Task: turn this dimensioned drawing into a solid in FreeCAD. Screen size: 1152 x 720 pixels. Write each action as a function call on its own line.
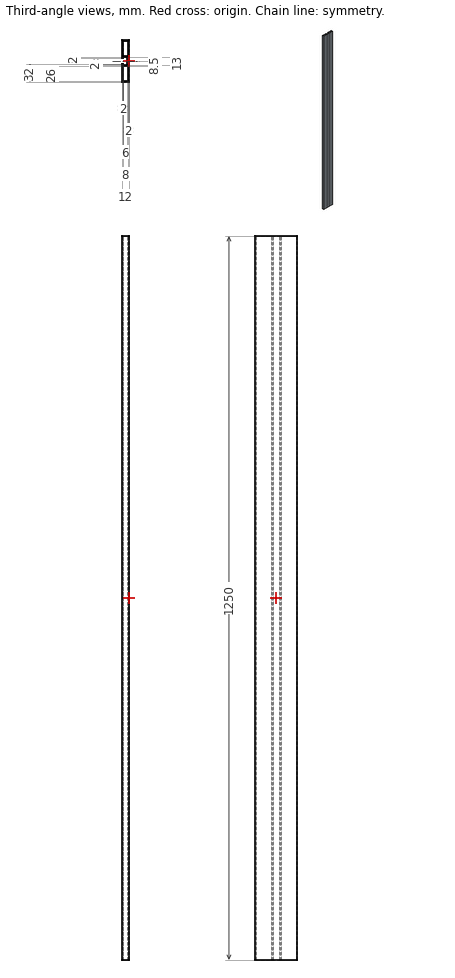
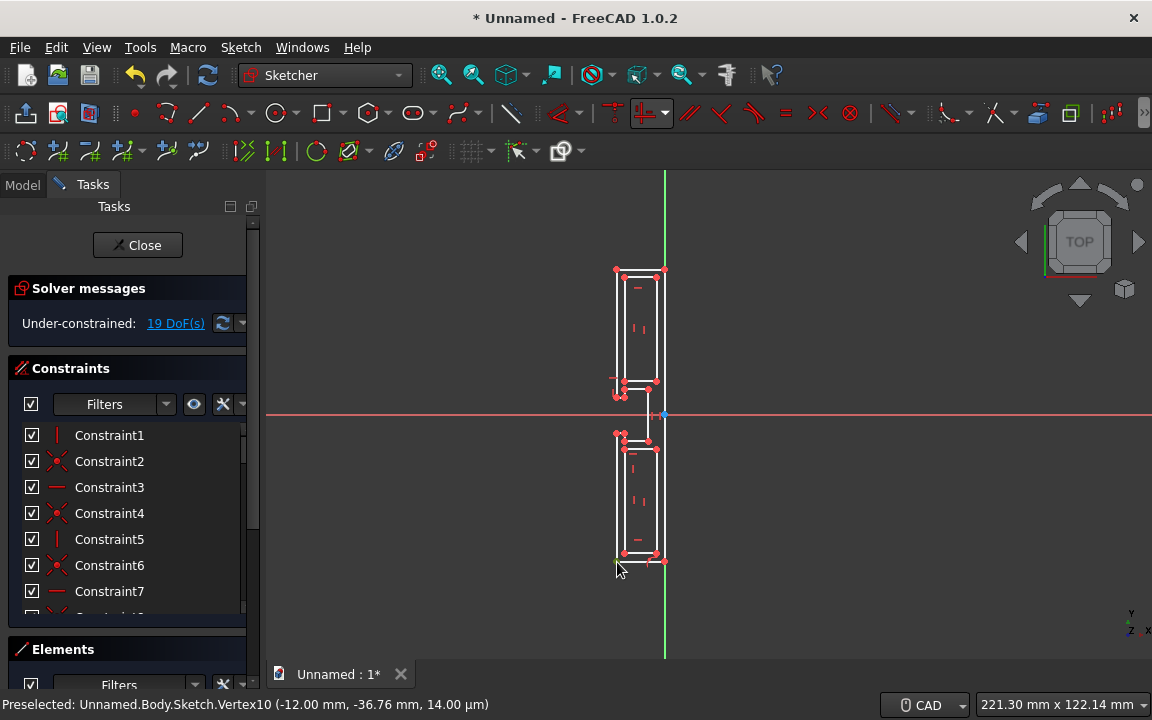
click(617, 270)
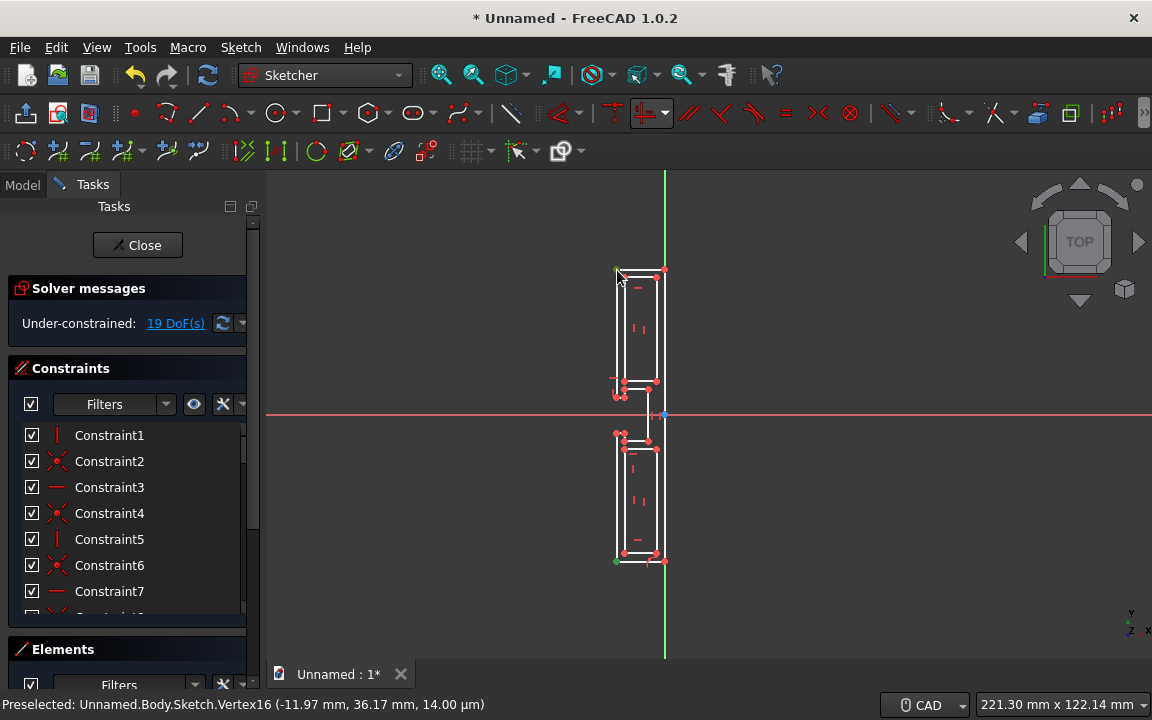
click(344, 415)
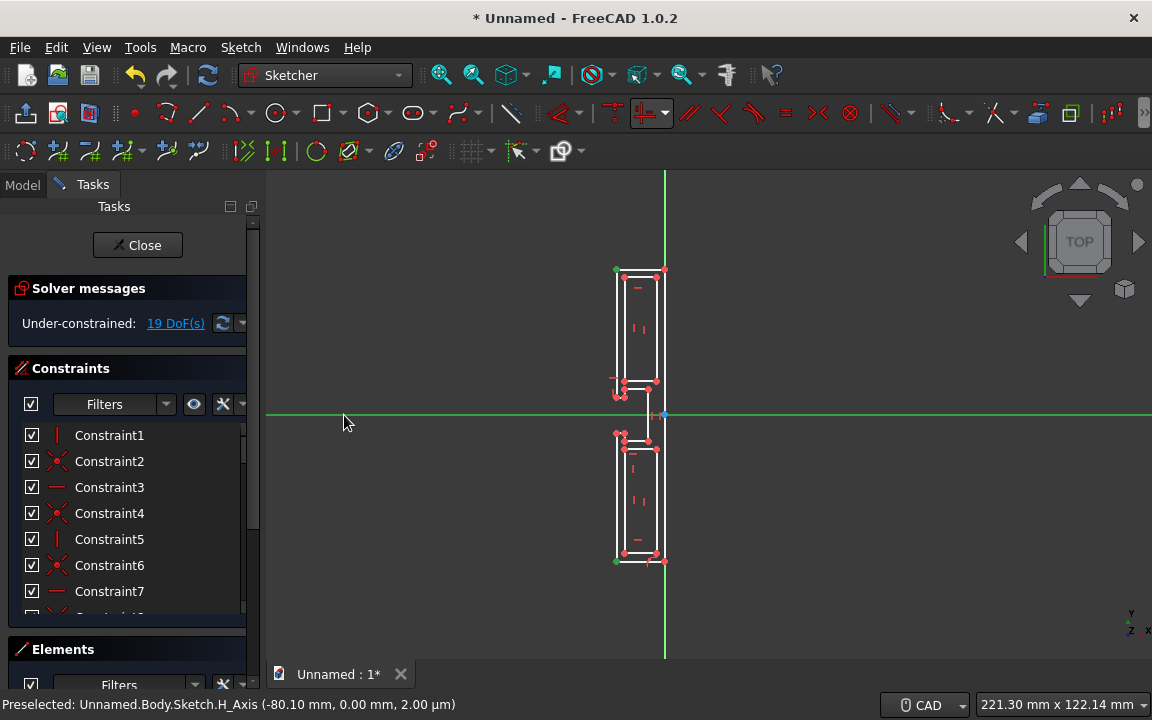
click(818, 114)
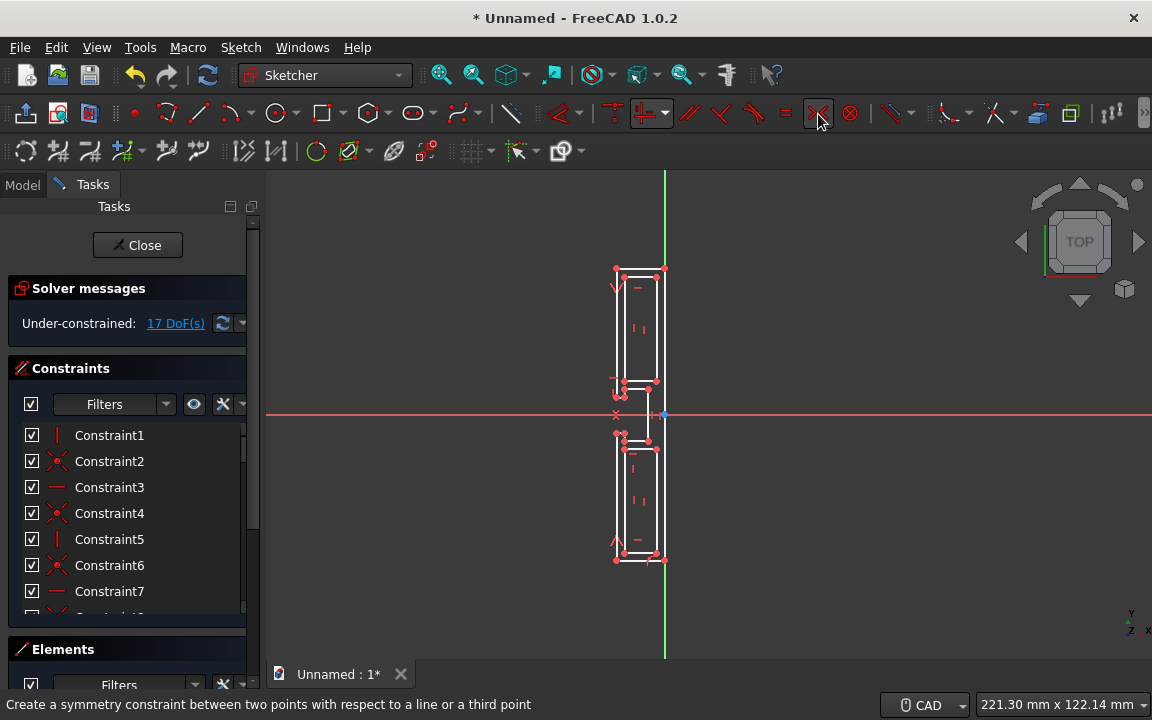
scroll(625, 433, up, 3)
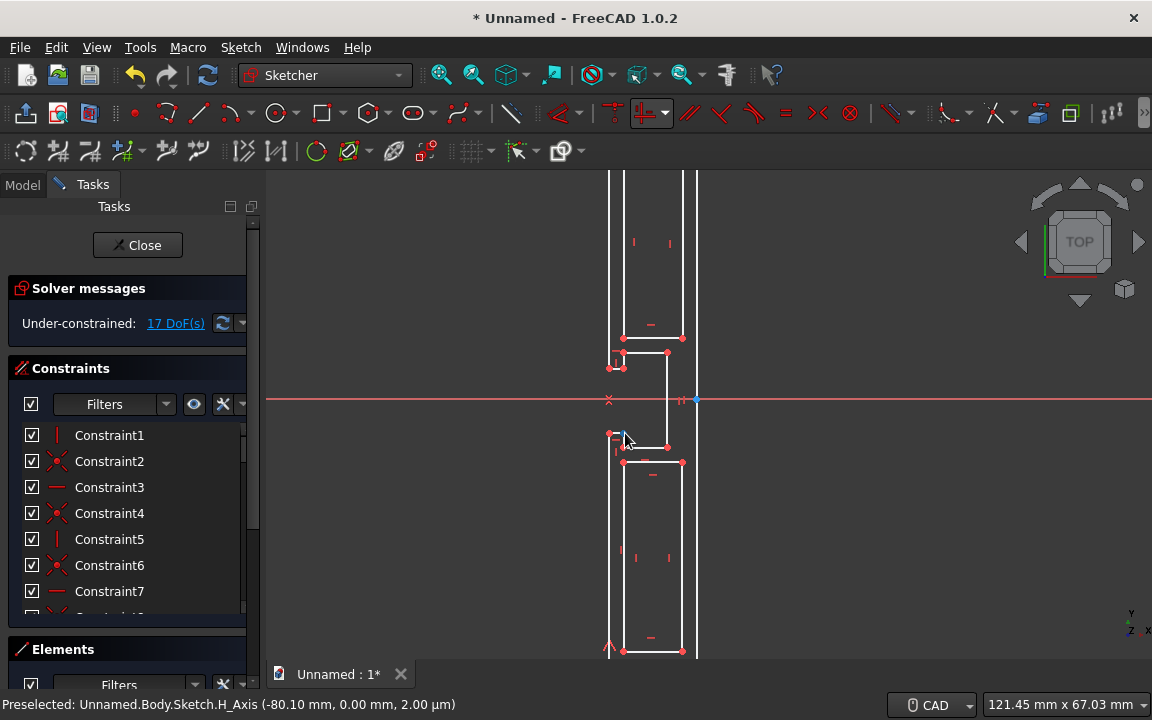
click(624, 433)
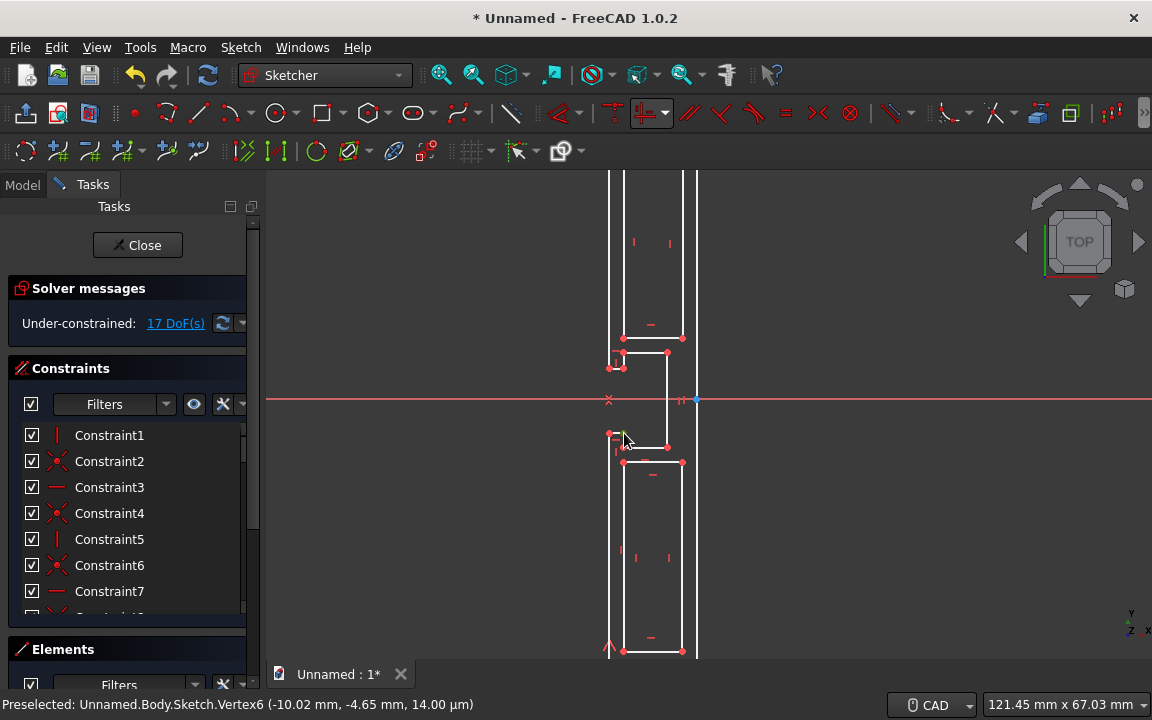
click(624, 369)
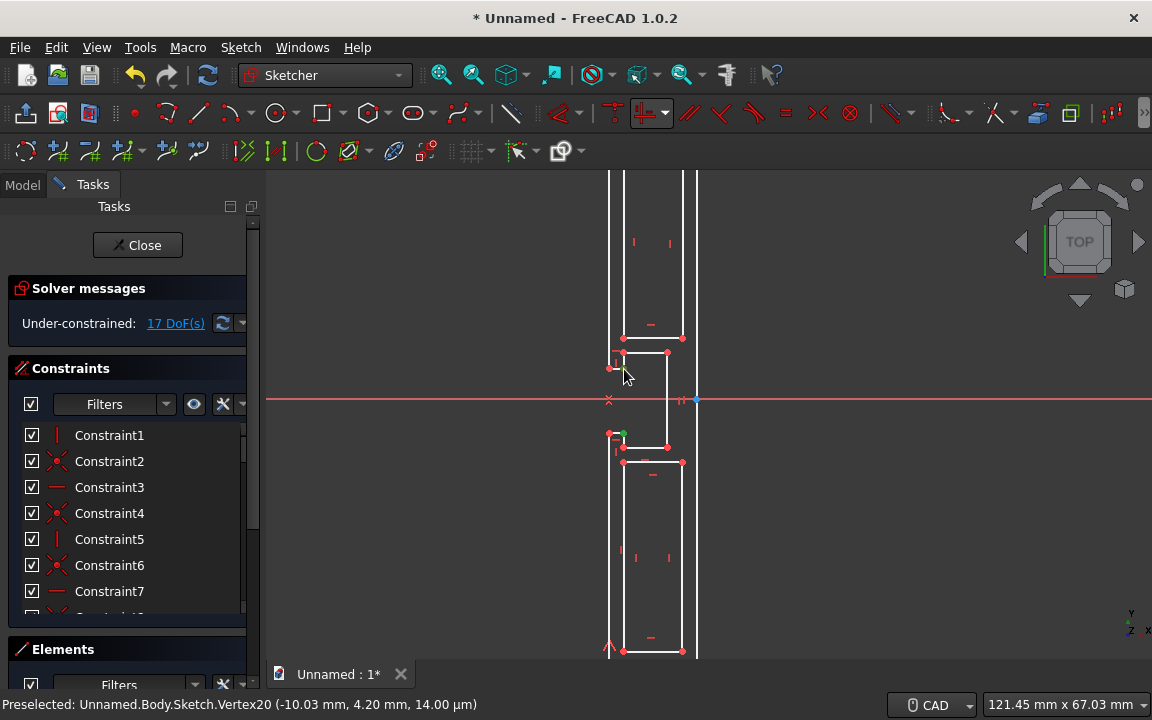
click(344, 399)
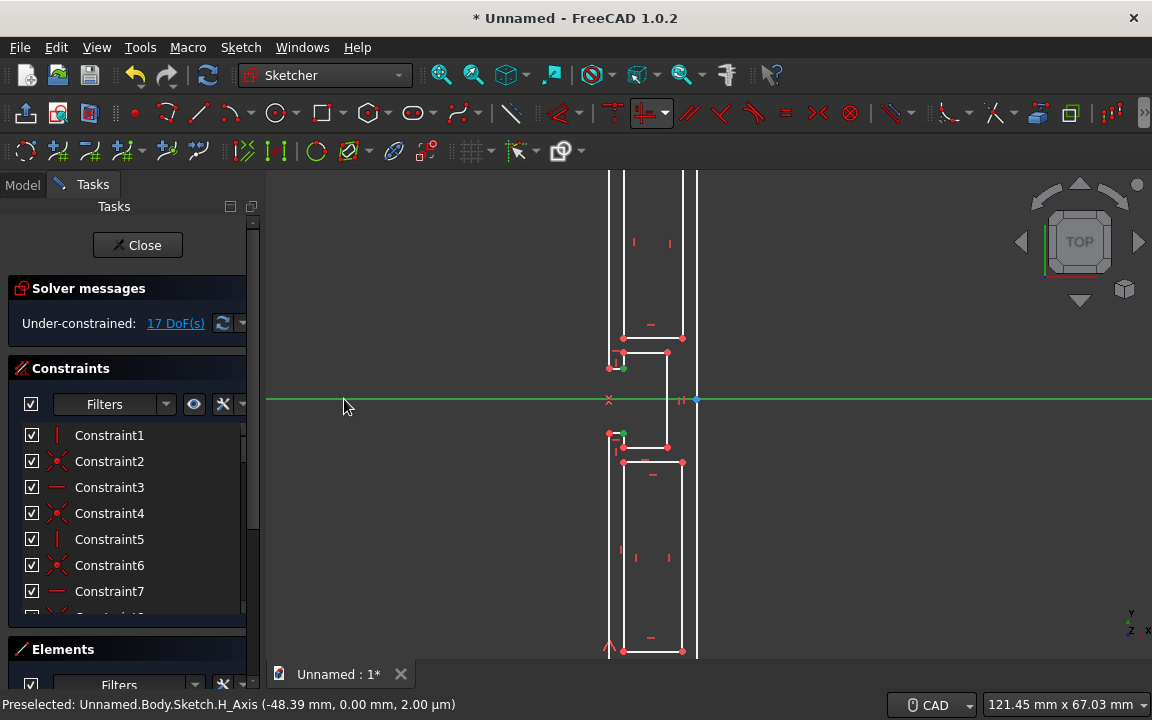
click(818, 114)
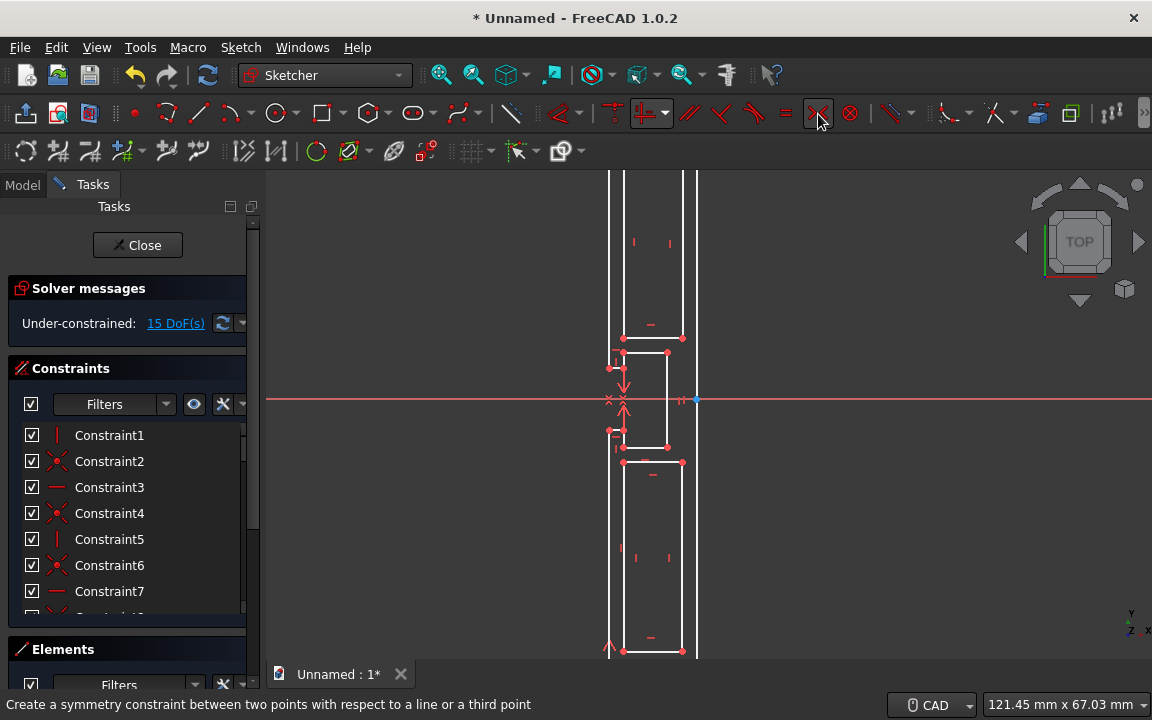
scroll(625, 433, down, 3)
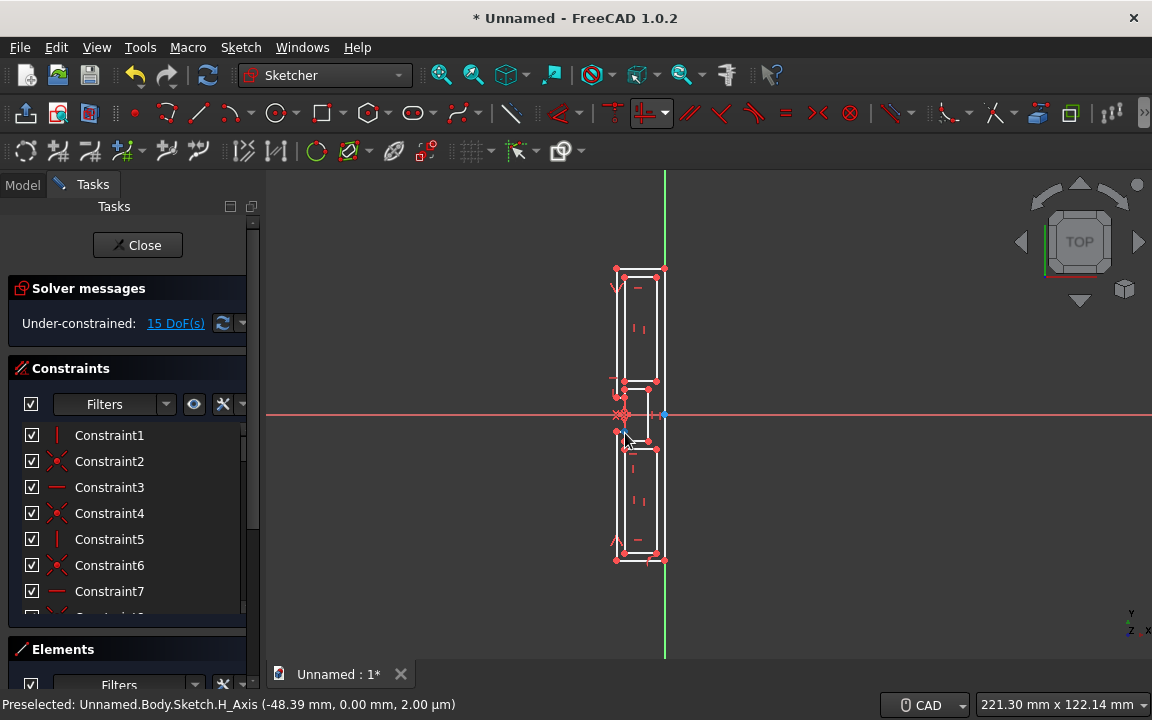
click(625, 553)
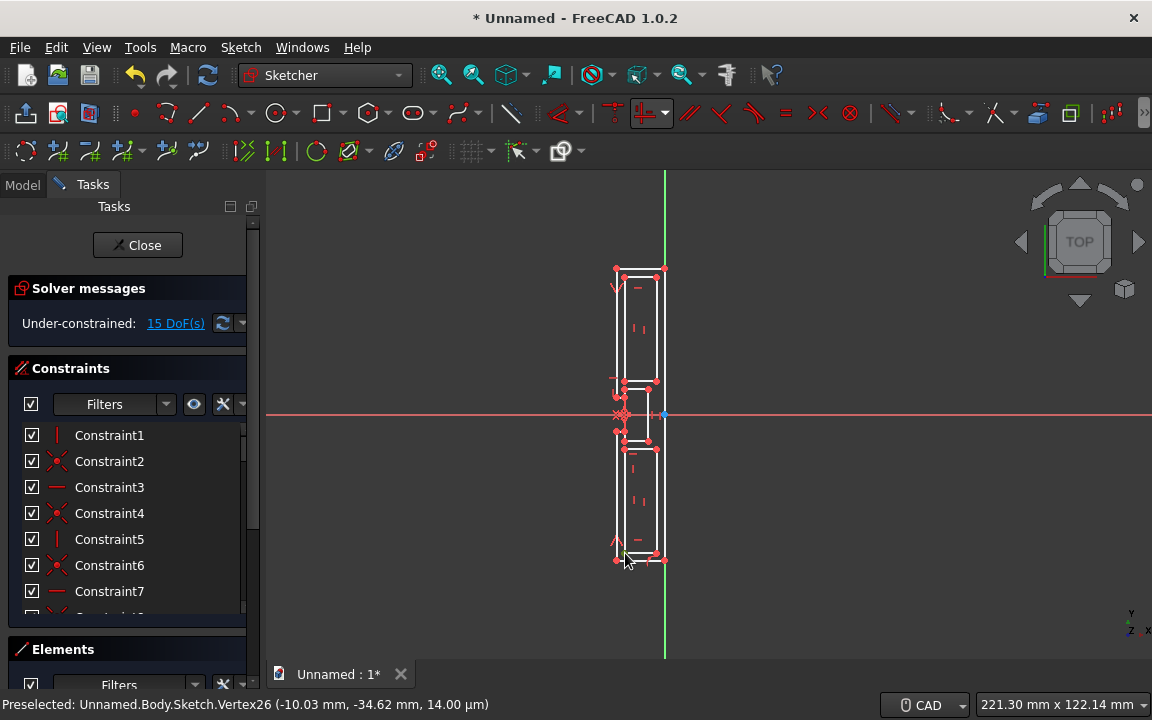
click(625, 277)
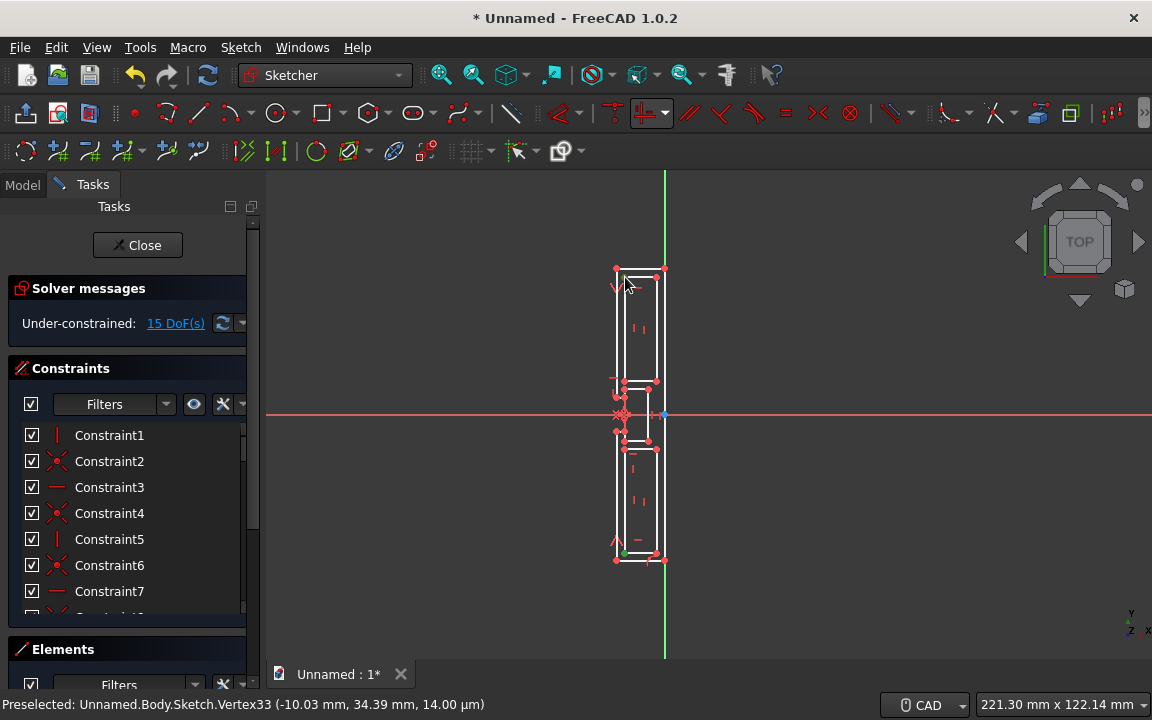
click(344, 415)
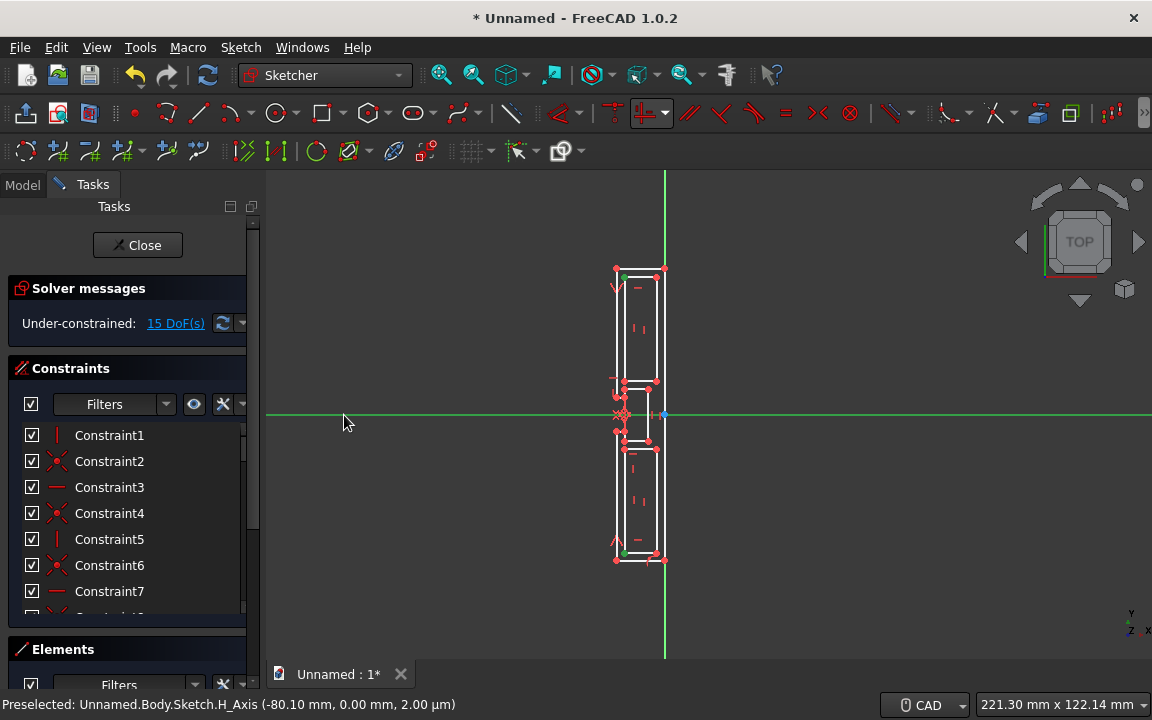
click(818, 114)